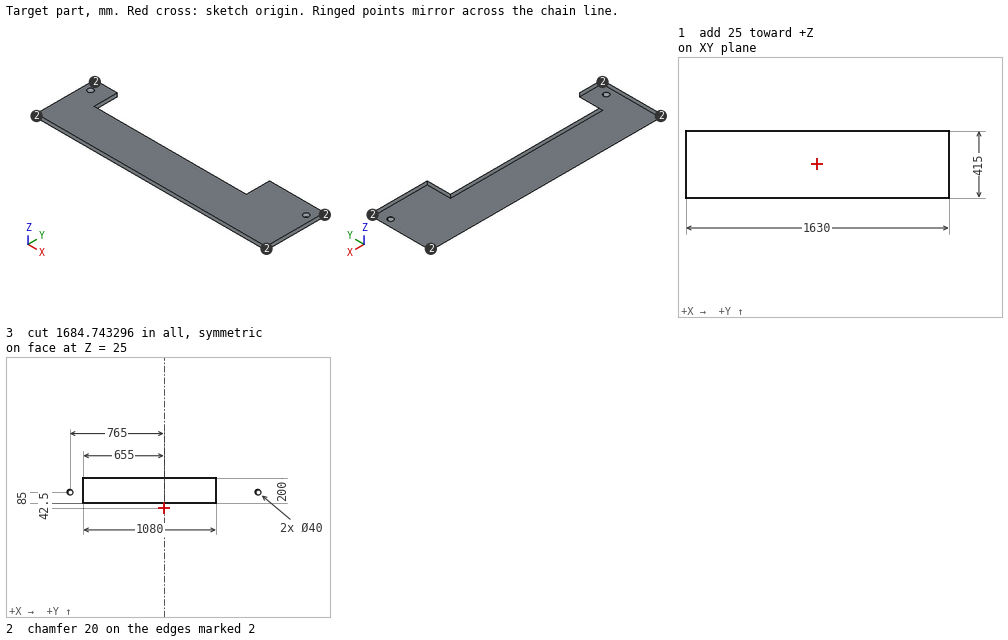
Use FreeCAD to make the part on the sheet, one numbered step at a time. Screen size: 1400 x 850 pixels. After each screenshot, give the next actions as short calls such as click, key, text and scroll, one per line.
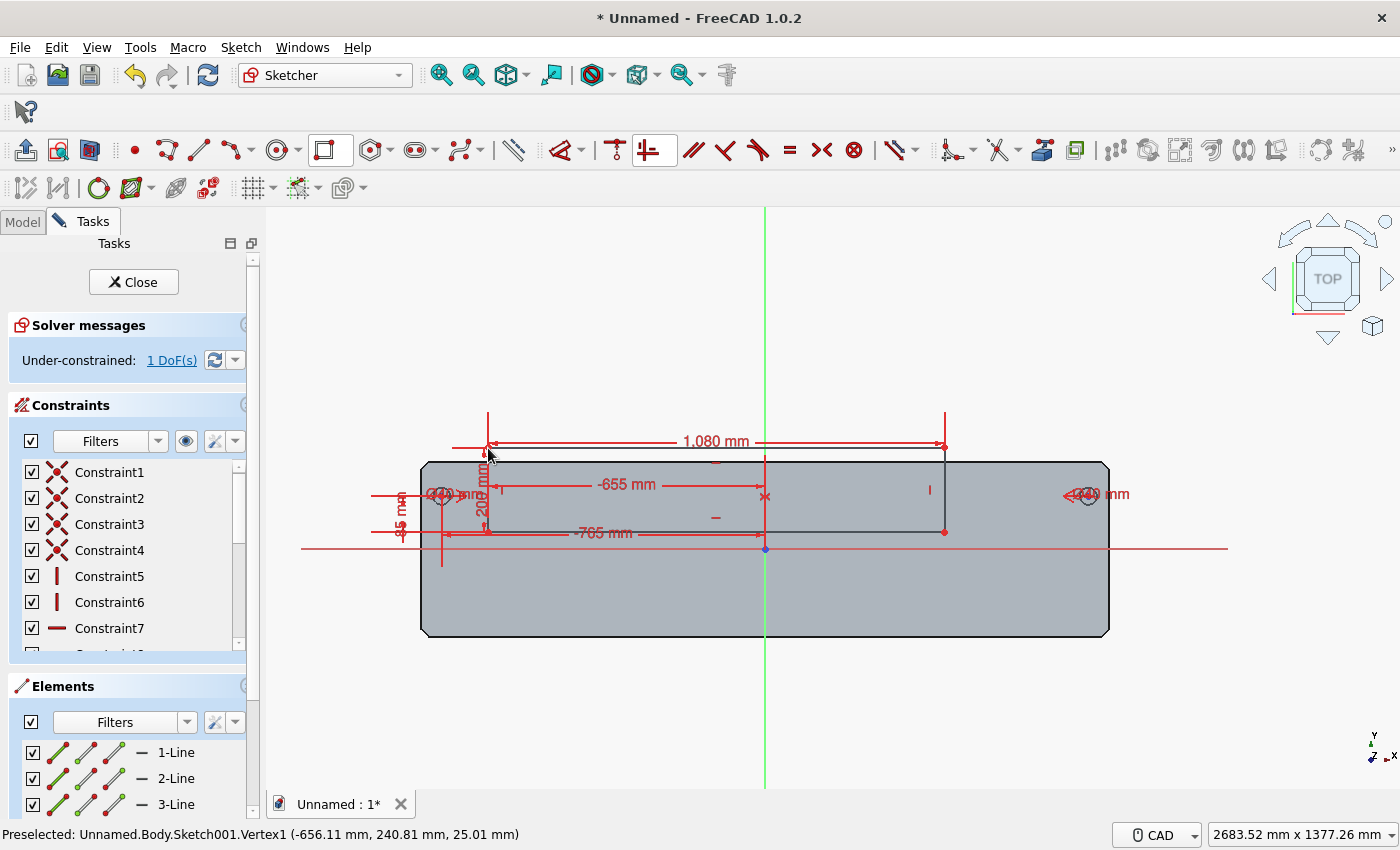
scroll(488, 532, up, 4)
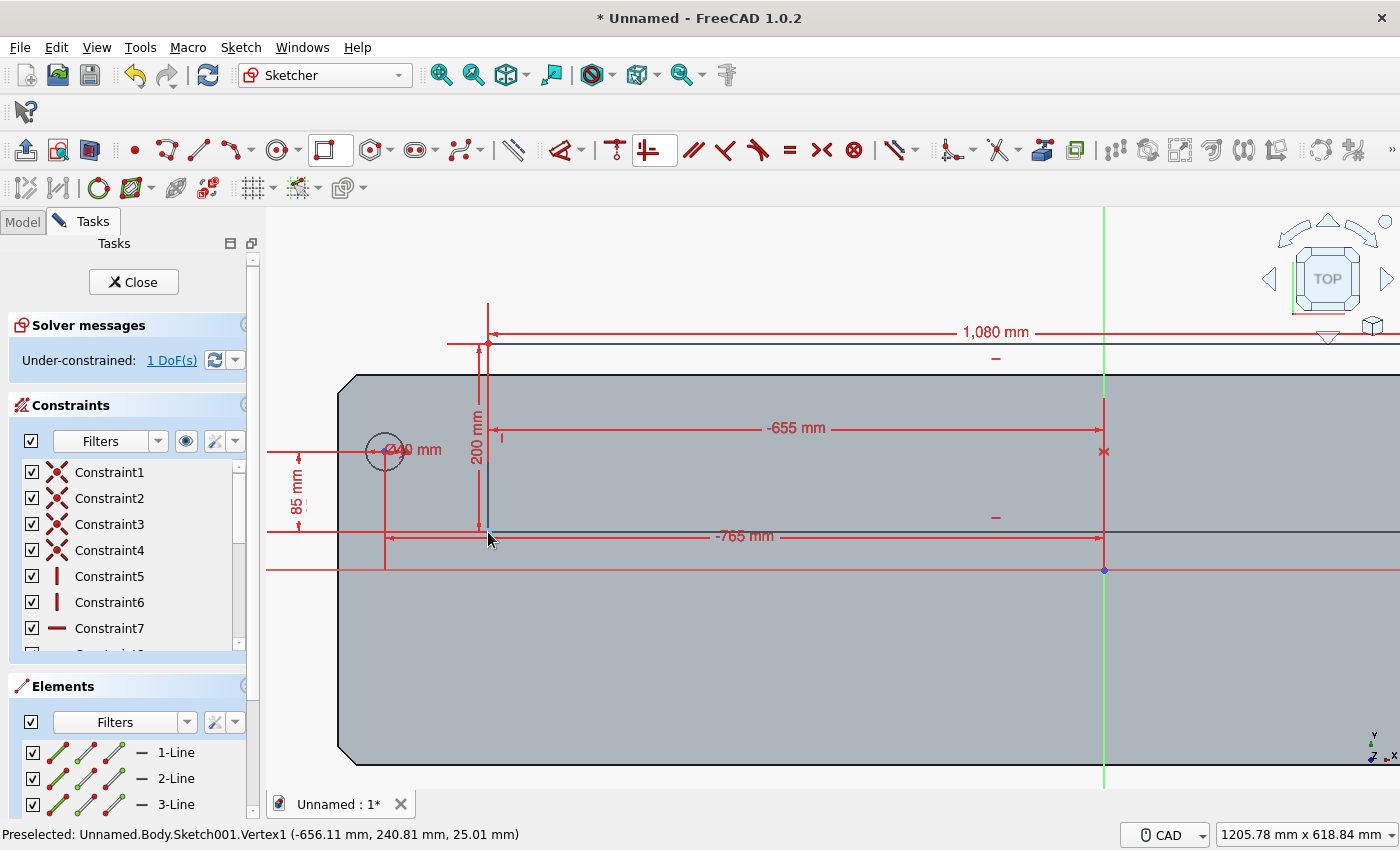
click(488, 532)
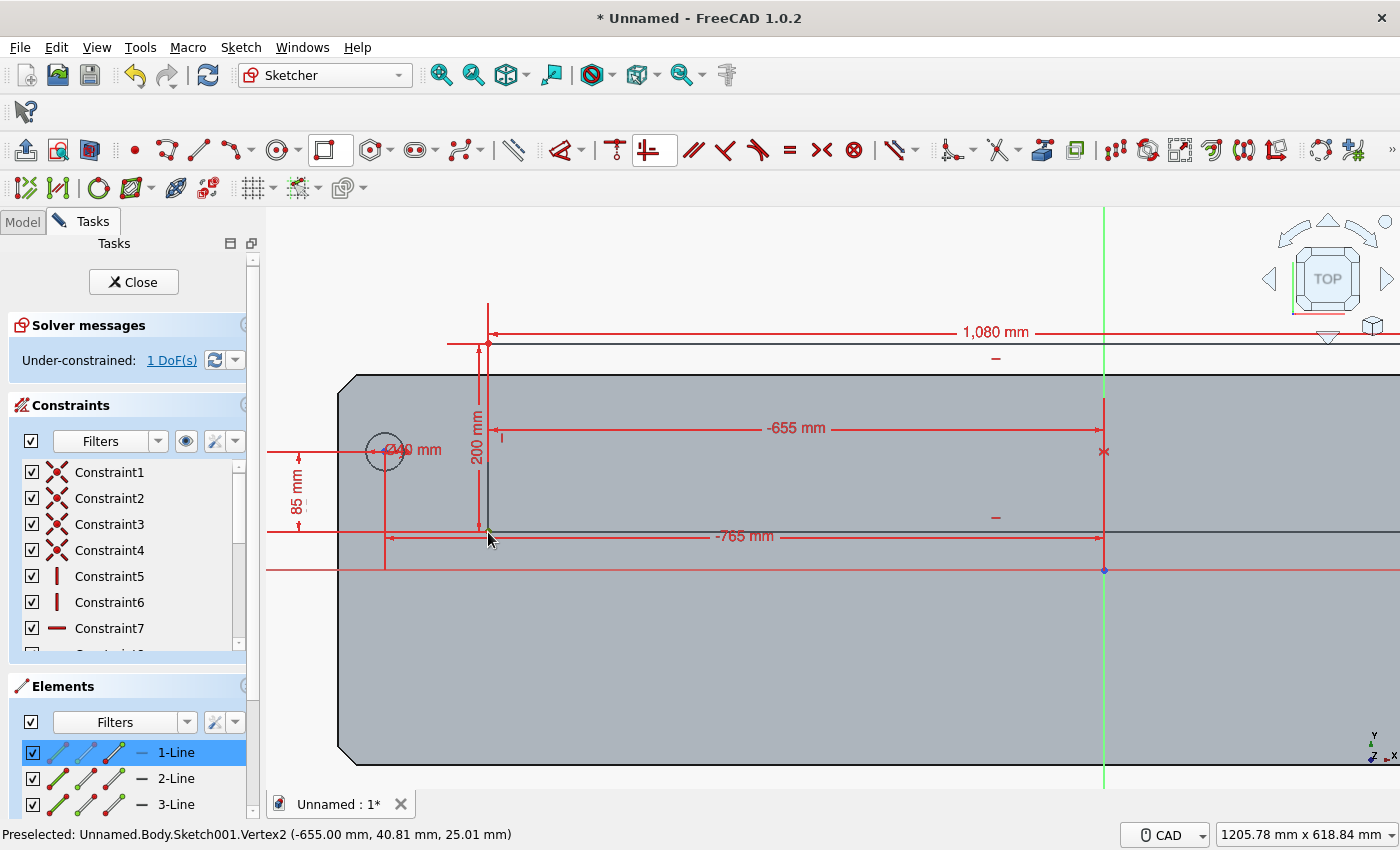
click(584, 150)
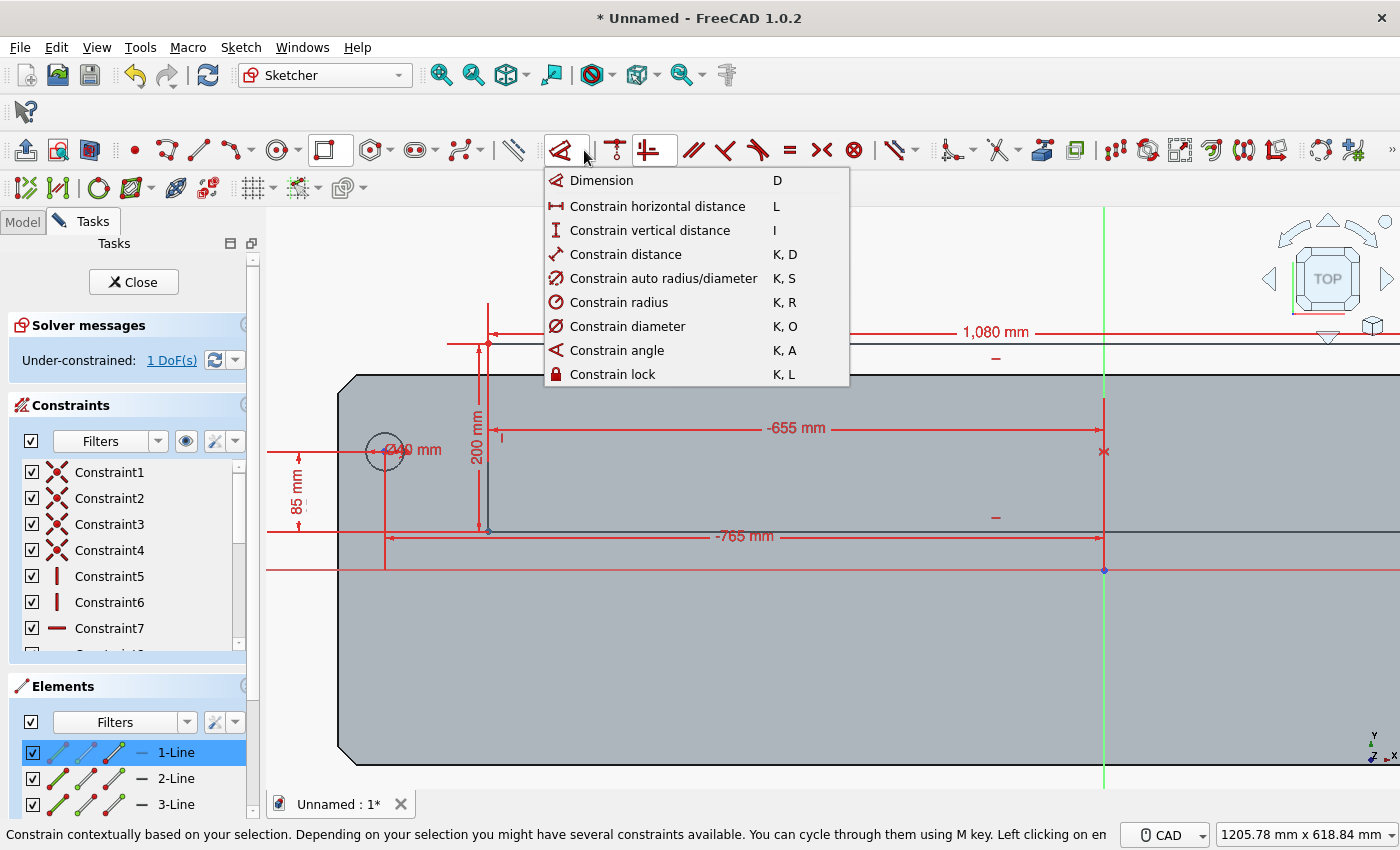
click(697, 230)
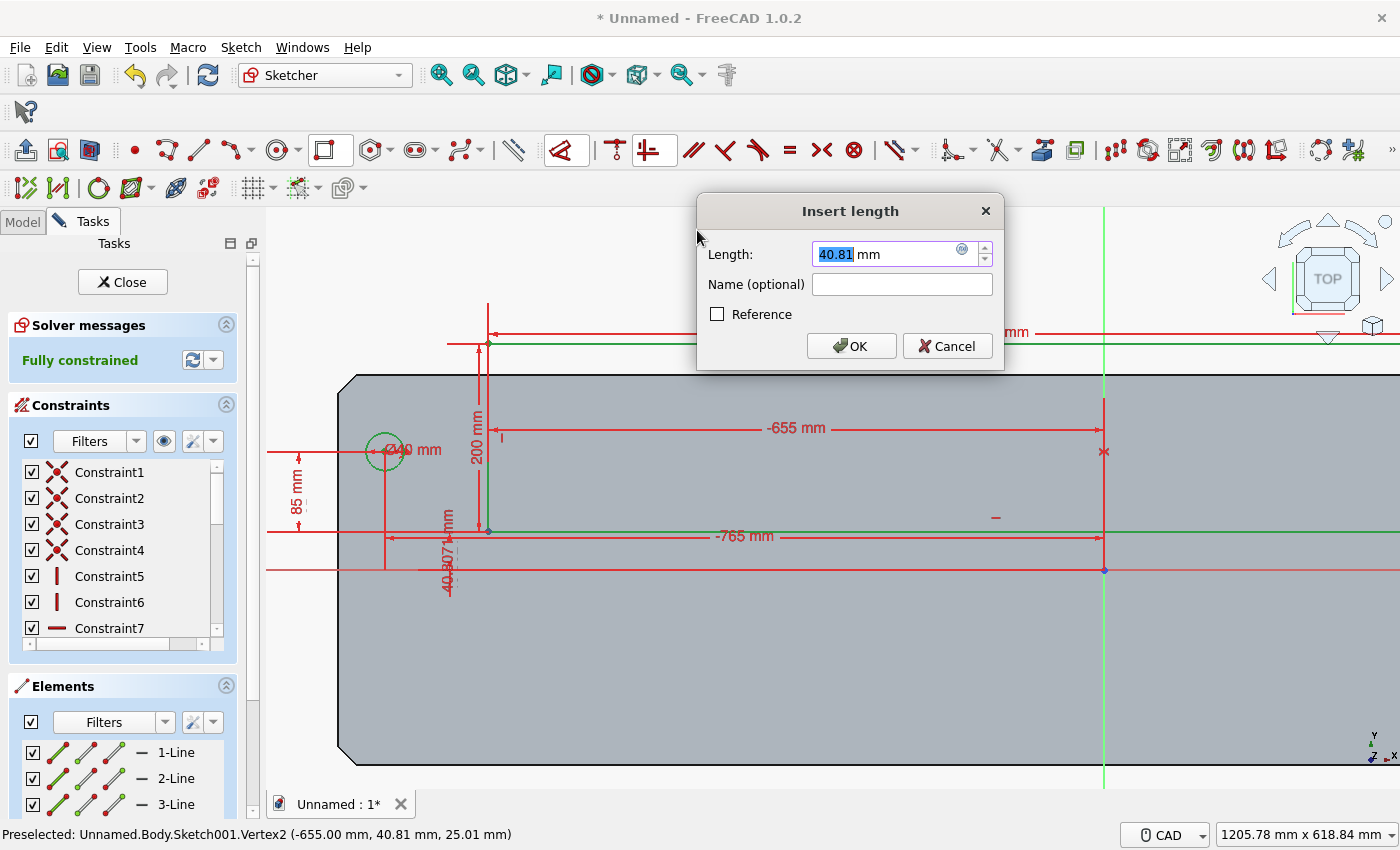
text(42.5)
key(Return)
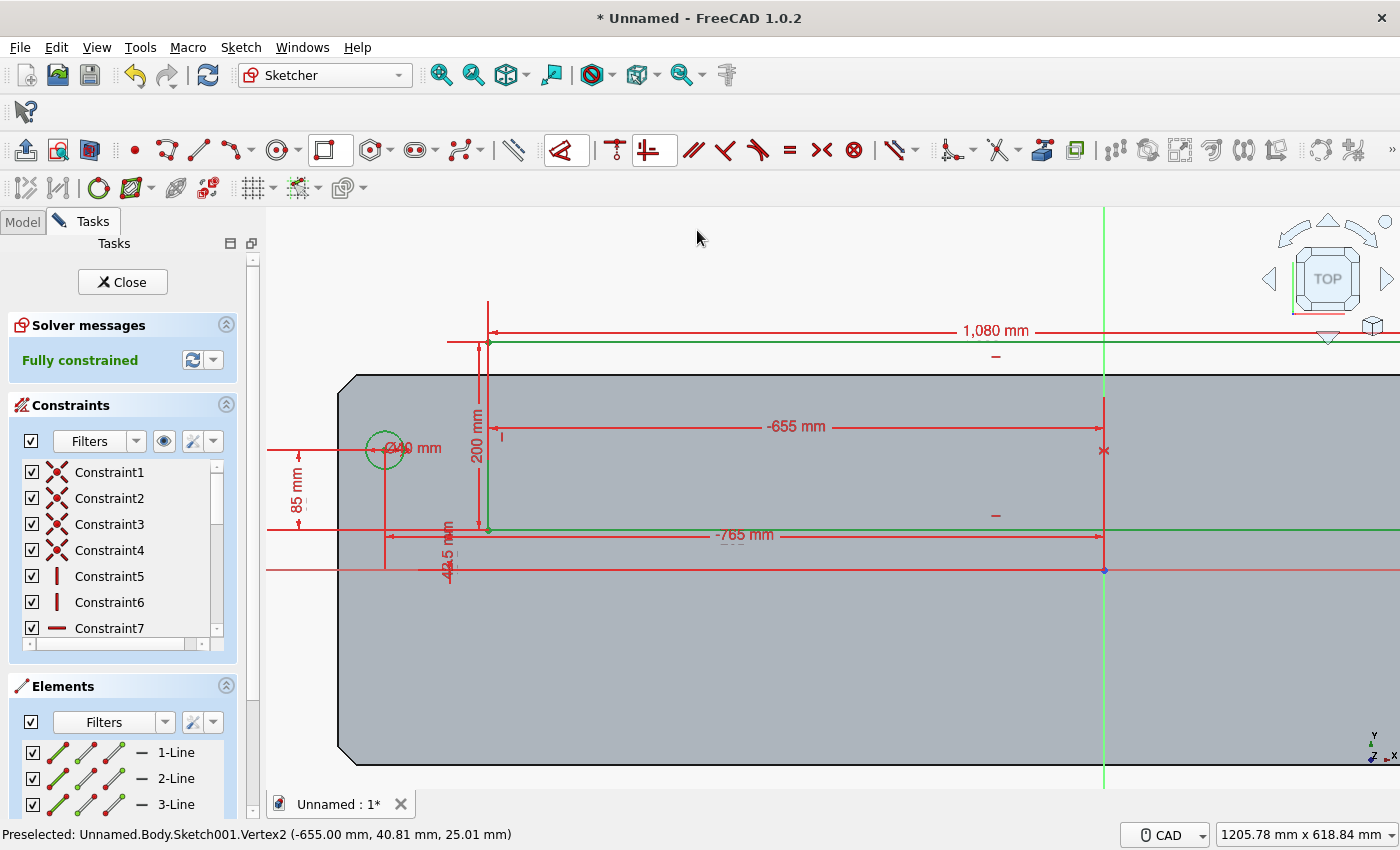
click(123, 282)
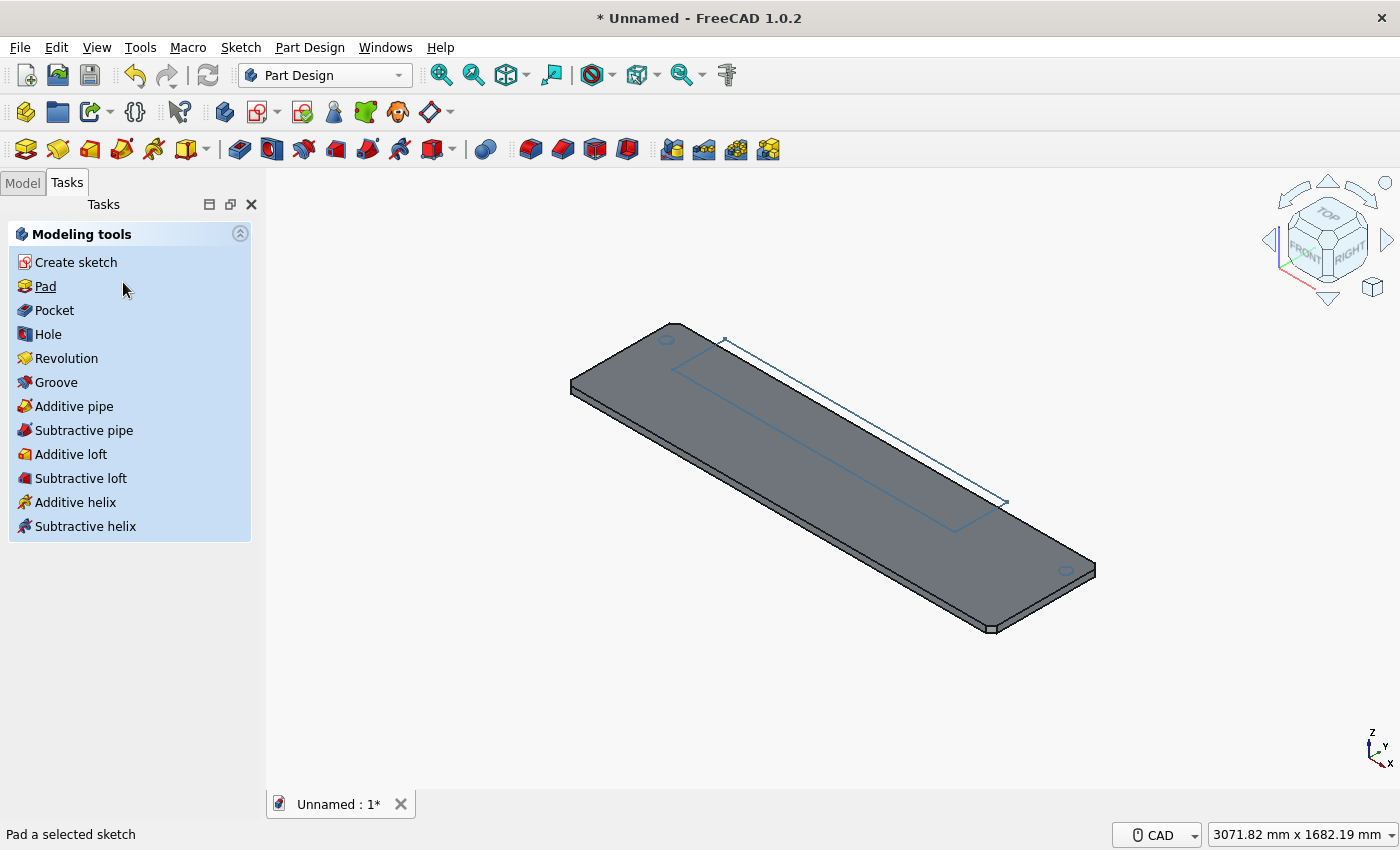
click(240, 150)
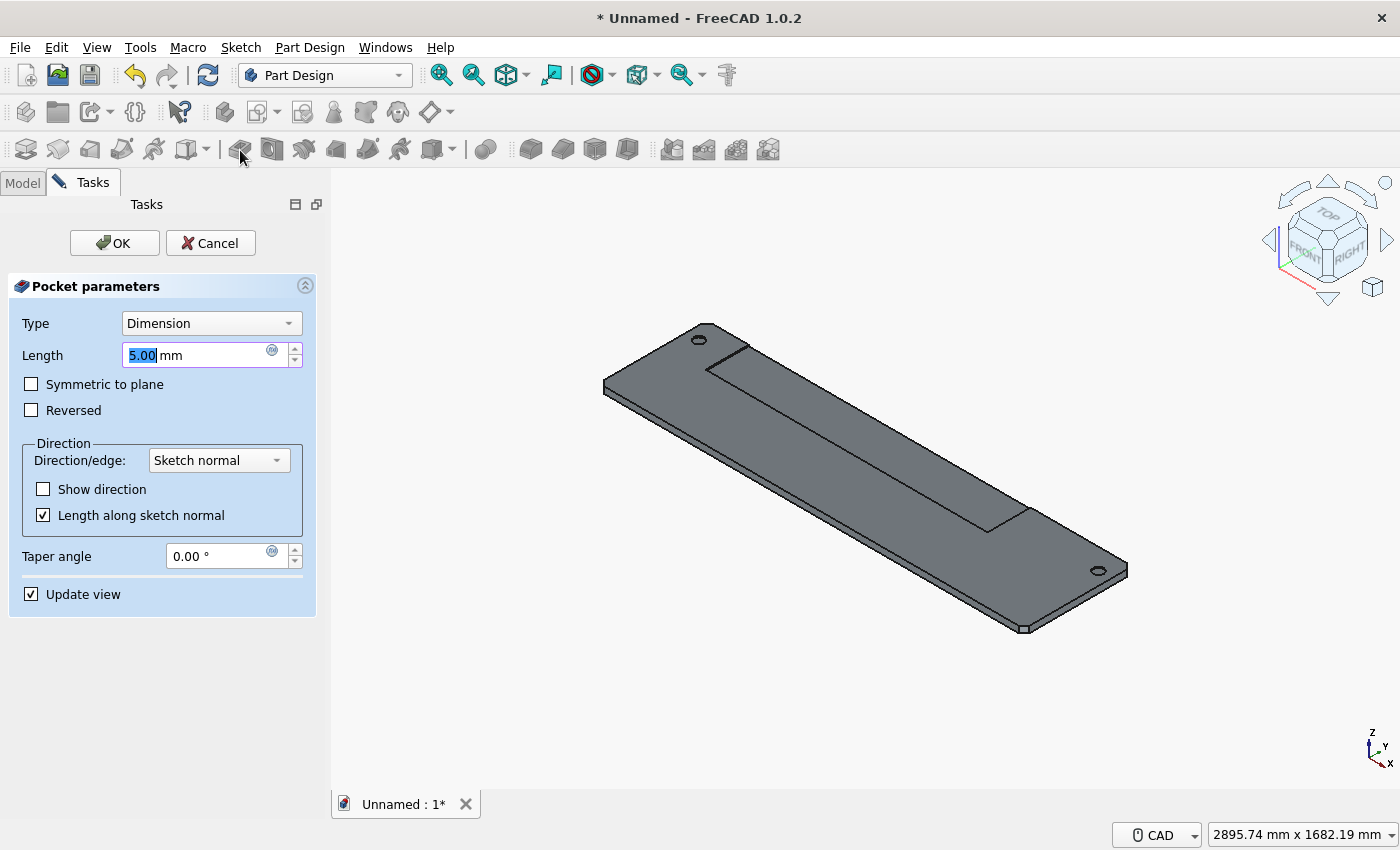
text(1684.743296)
key(Tab)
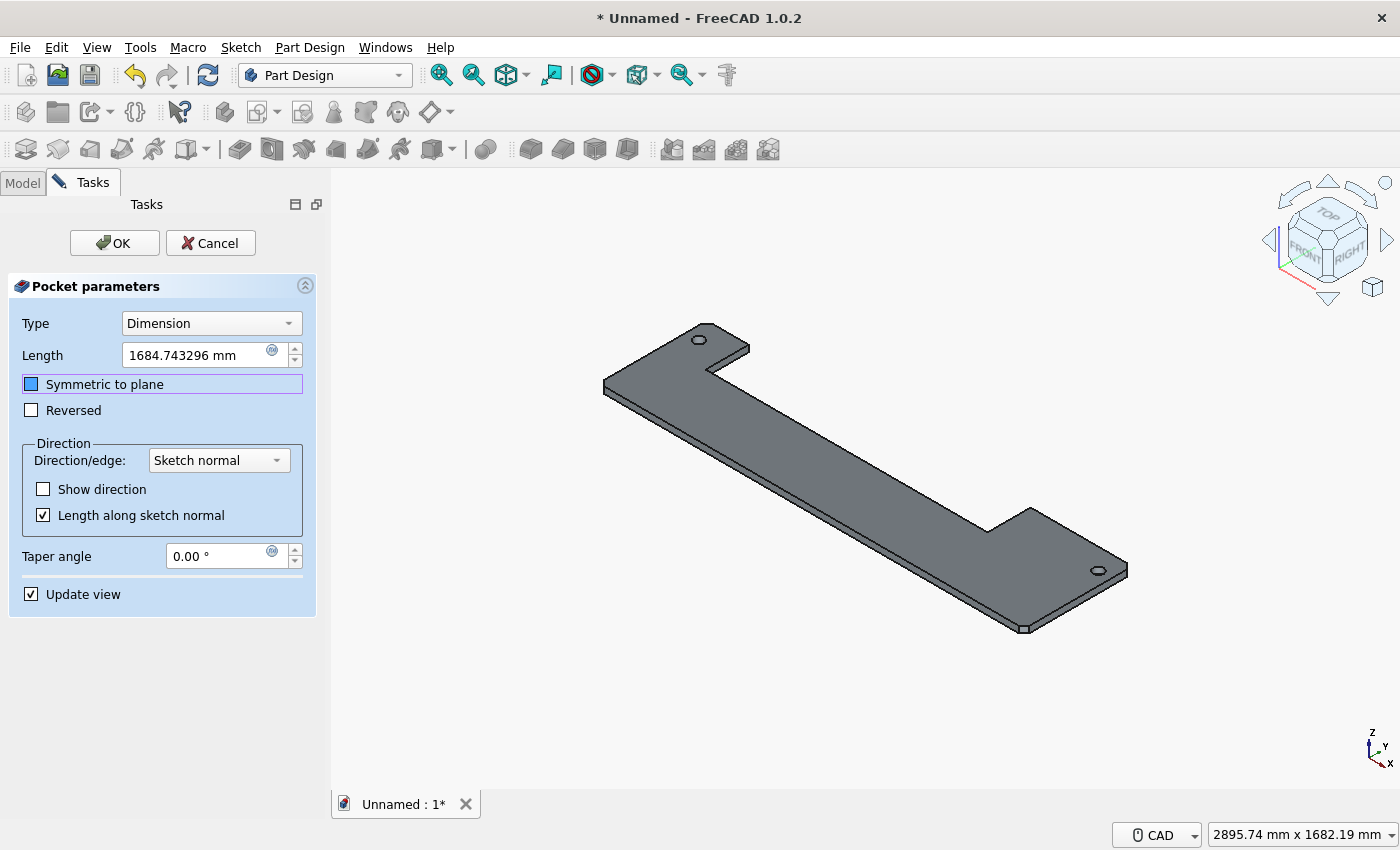
click(30, 384)